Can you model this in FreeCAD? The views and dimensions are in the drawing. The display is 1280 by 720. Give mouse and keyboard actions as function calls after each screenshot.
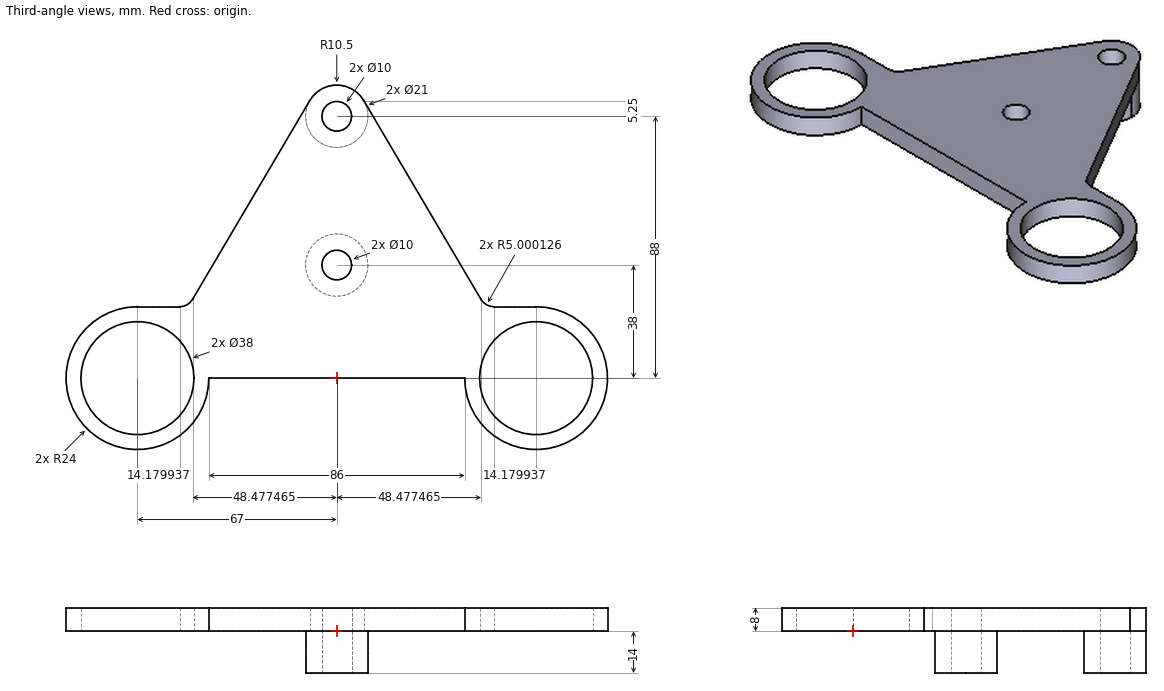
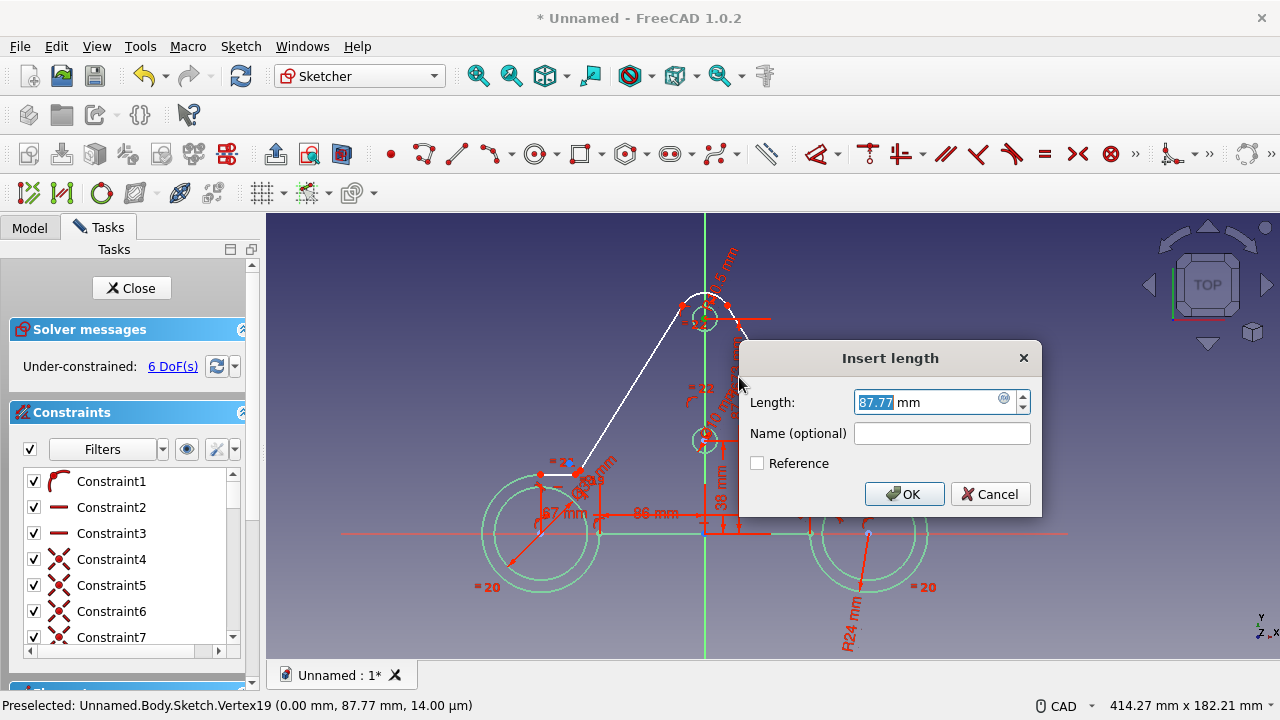
text(88)
key(Return)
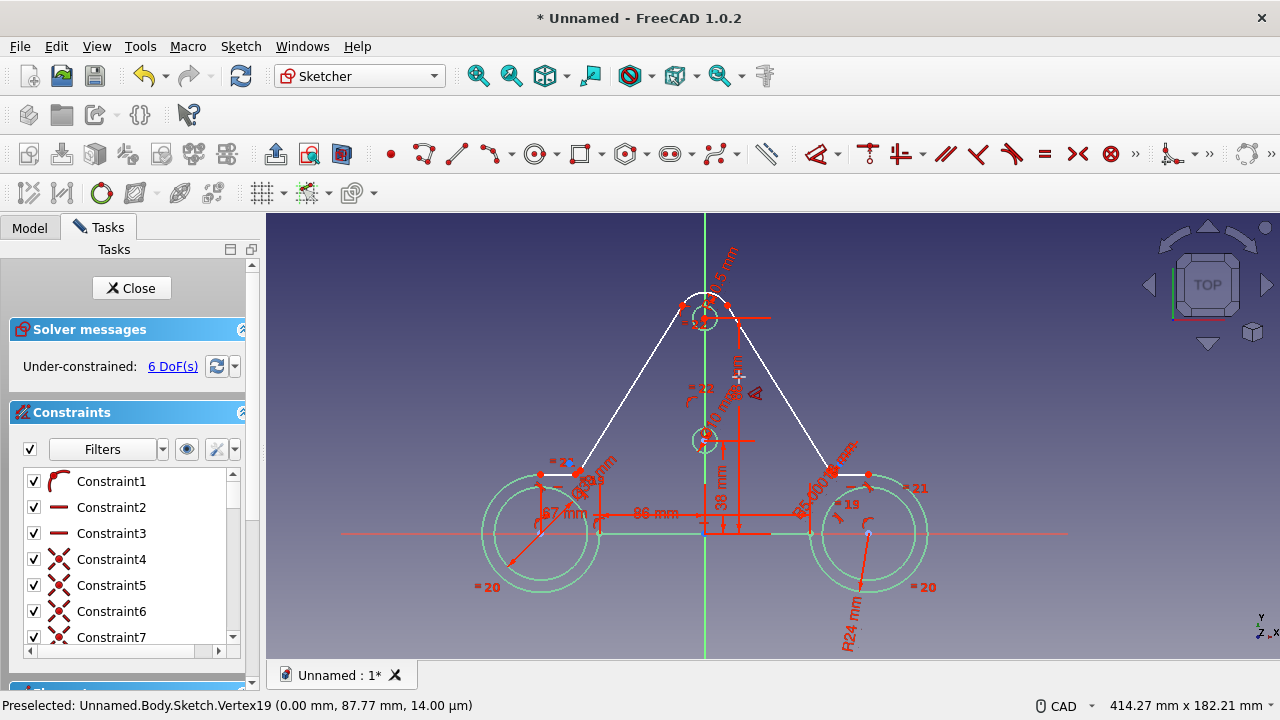
scroll(727, 306, up, 6)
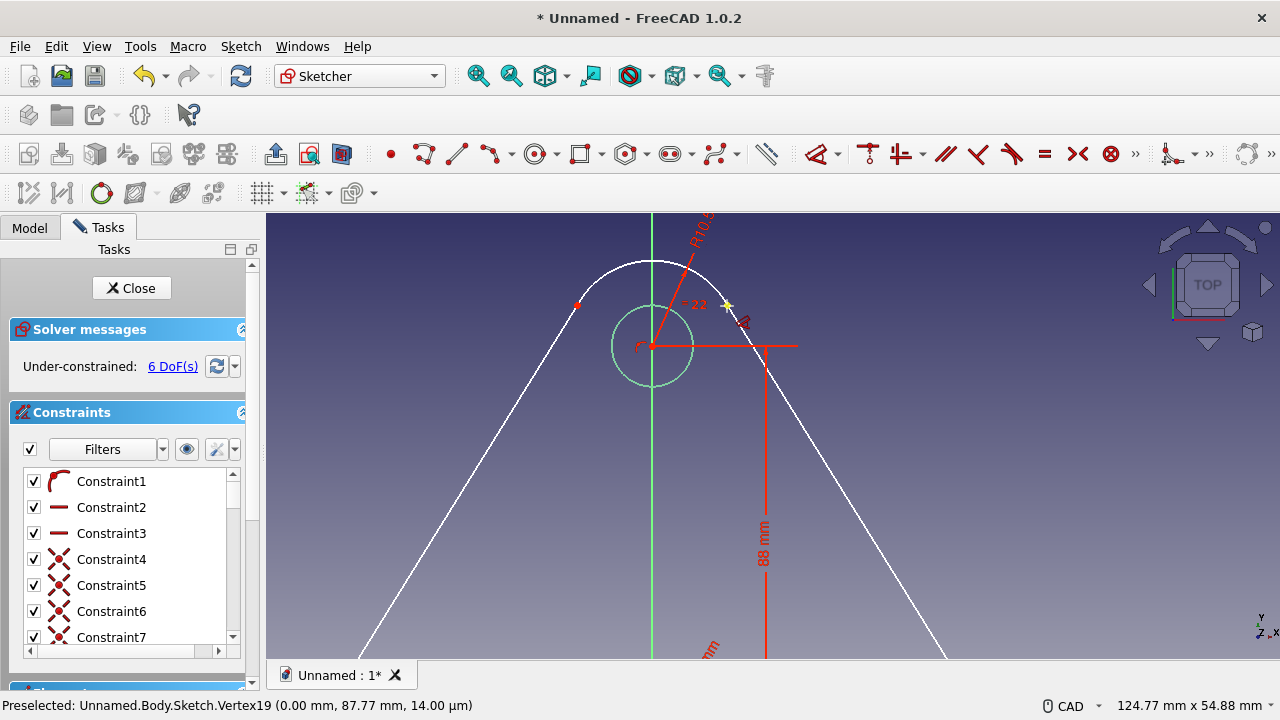
click(727, 305)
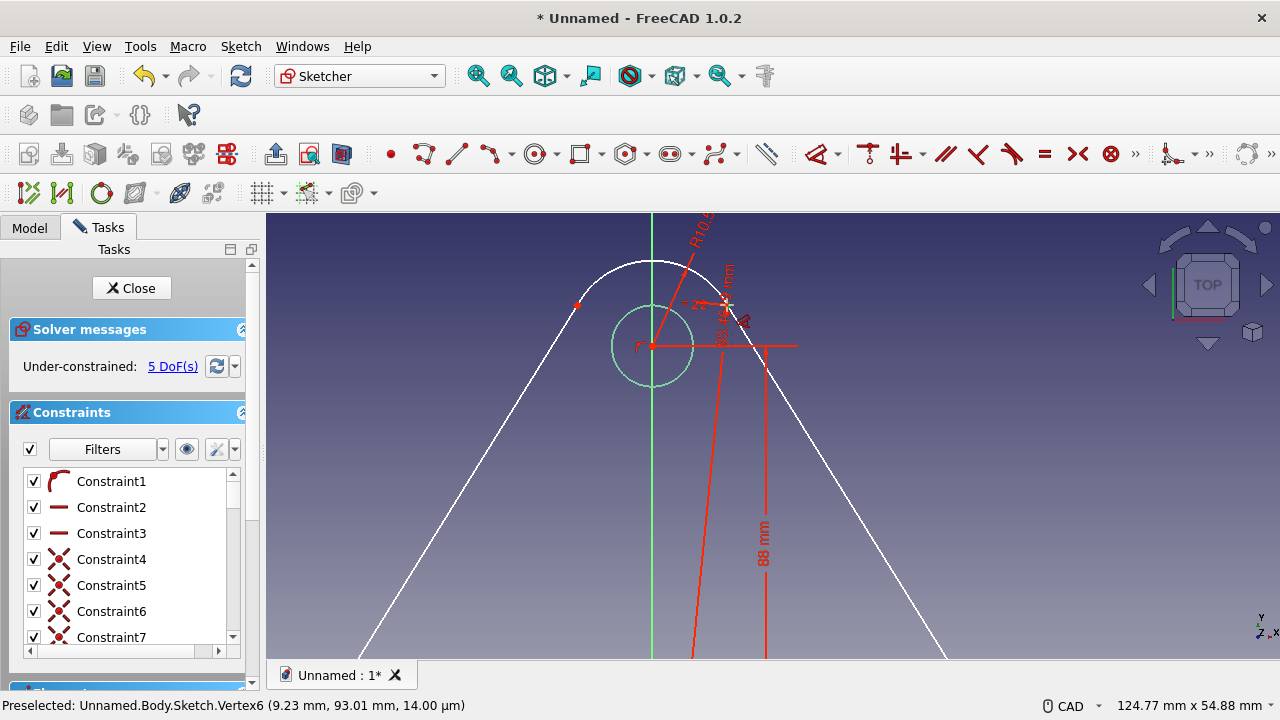
click(652, 346)
click(761, 326)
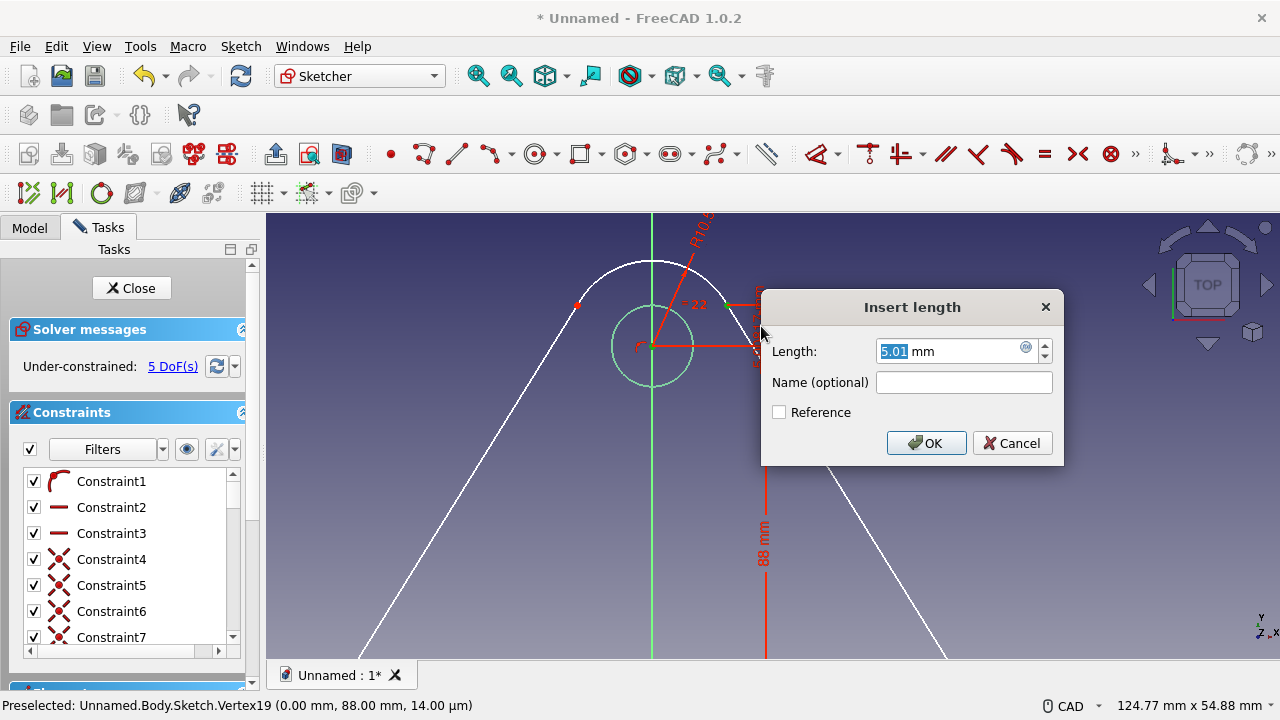
text(5.25)
key(Return)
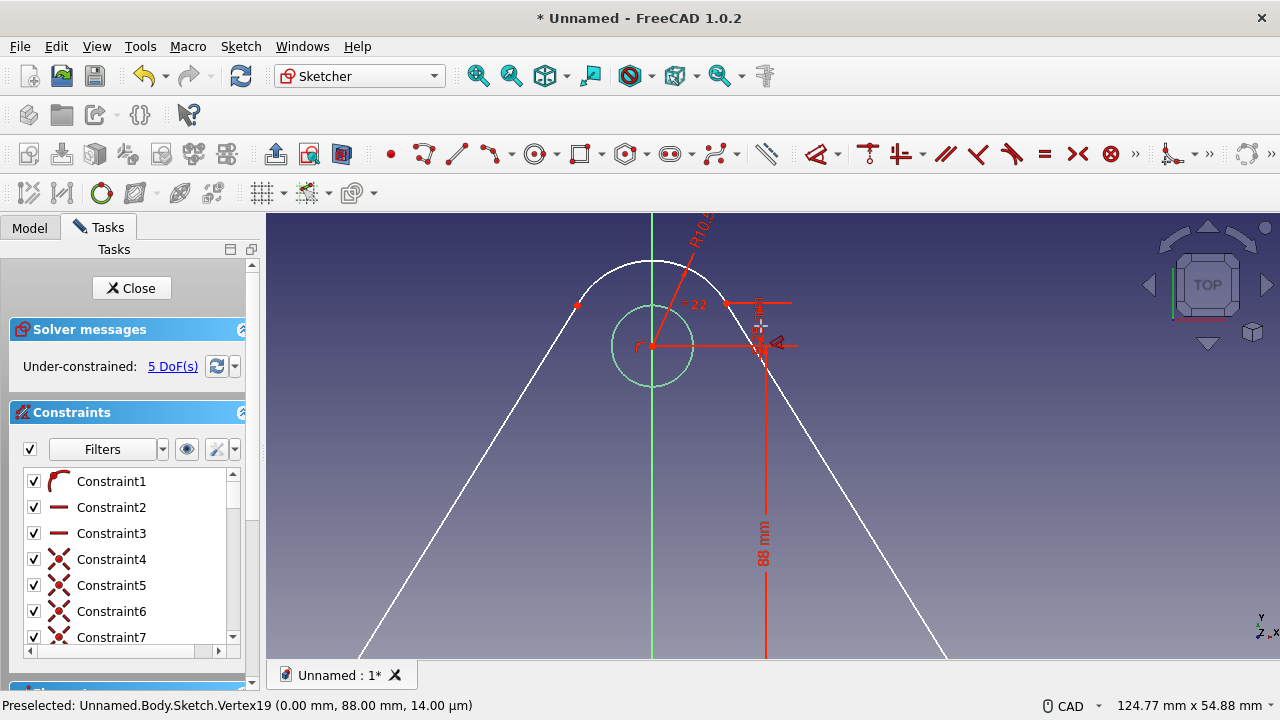
click(577, 305)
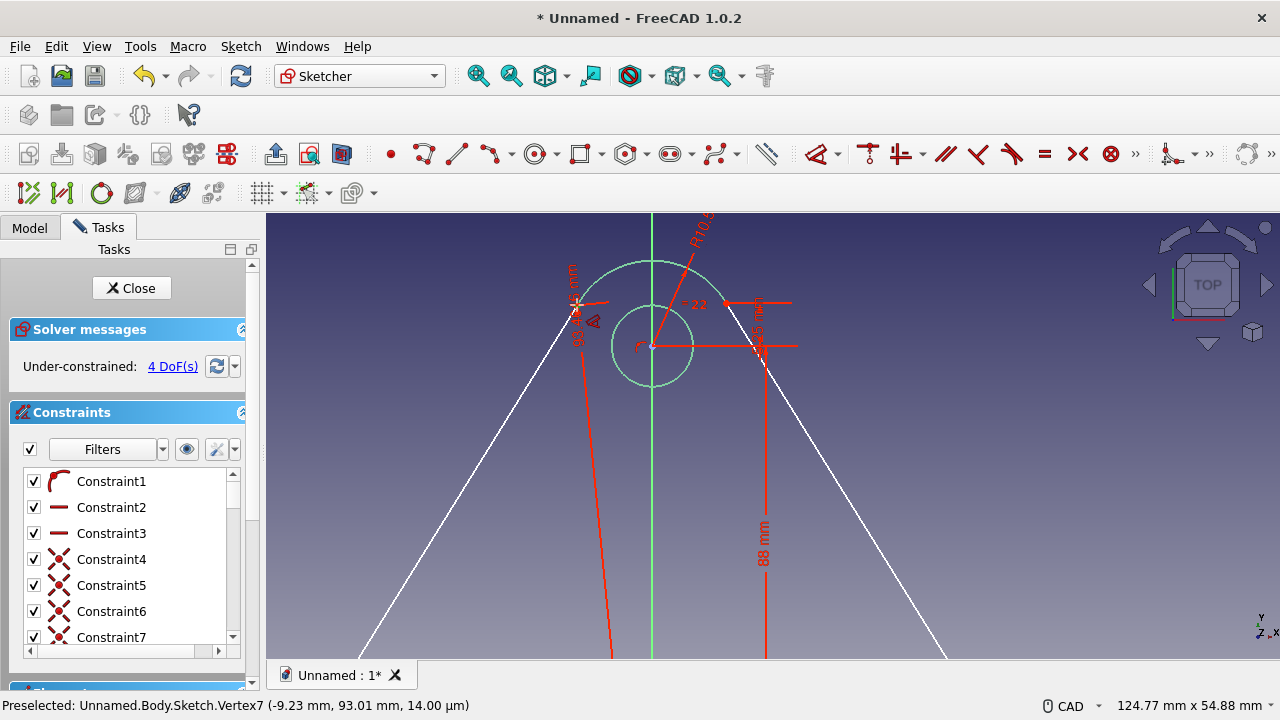
click(652, 346)
click(543, 326)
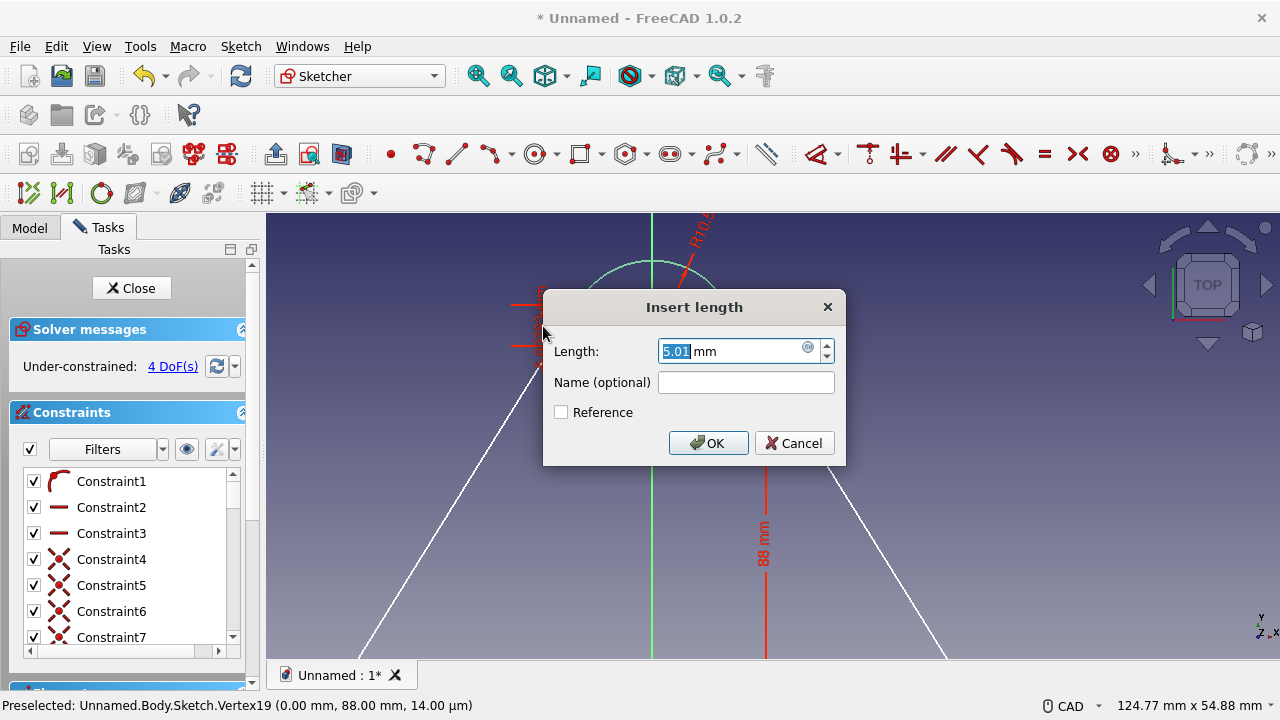
text(5.25)
key(Return)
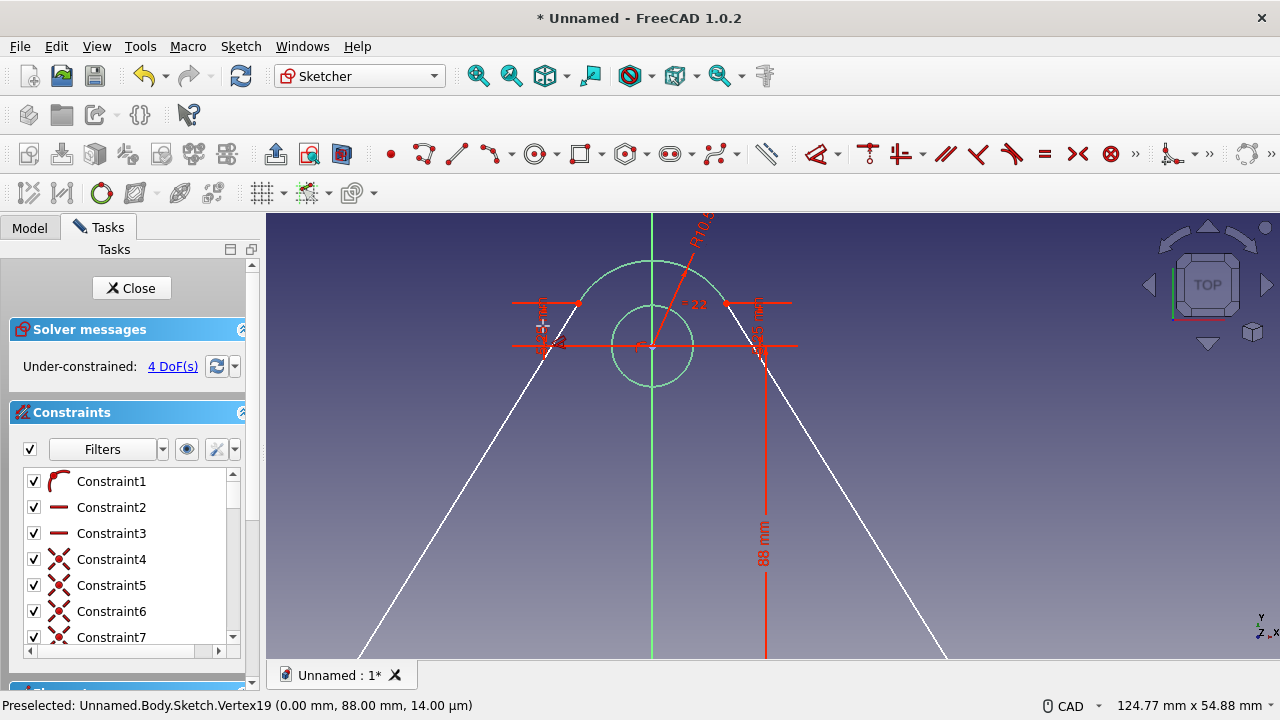
scroll(727, 306, down, 6)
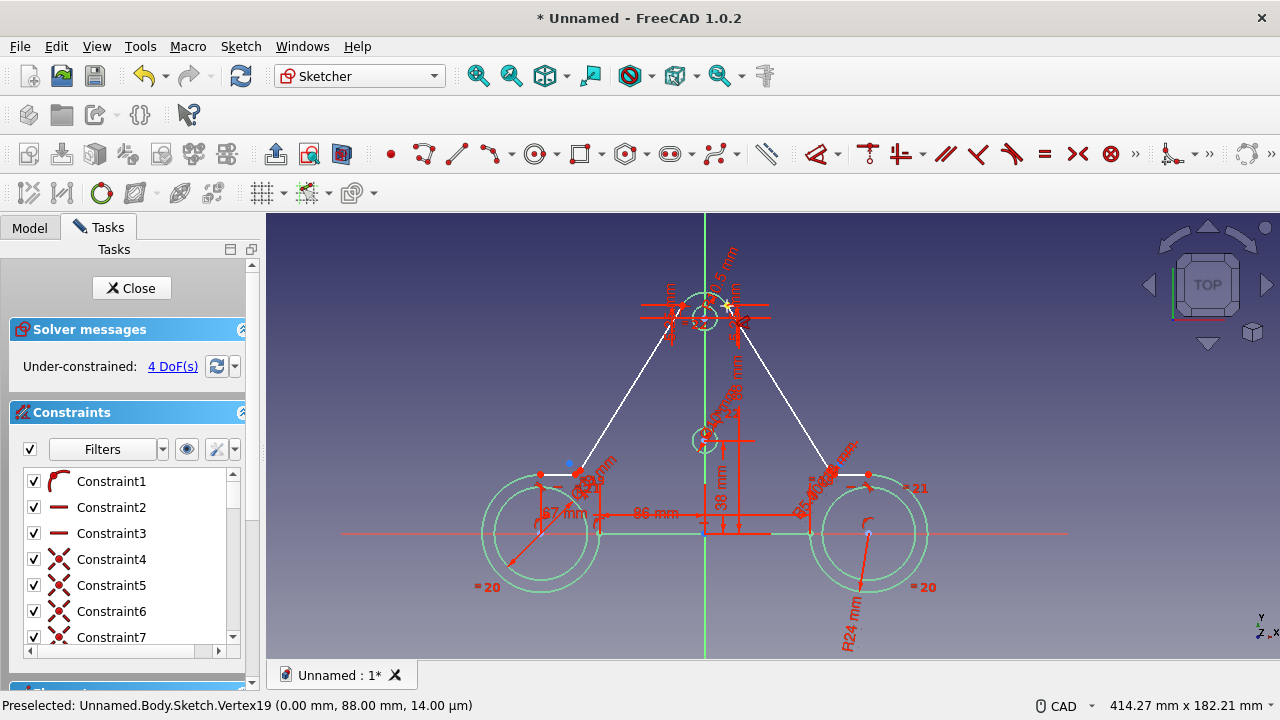
scroll(859, 475, up, 2)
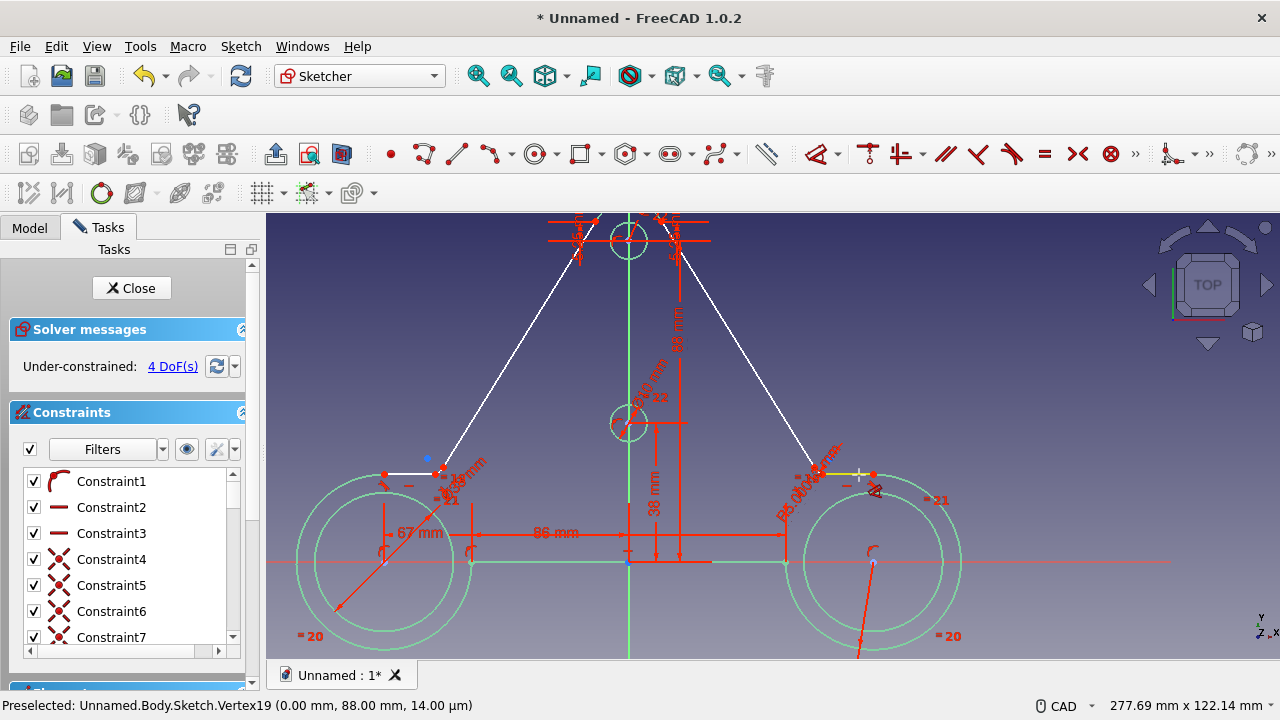
click(858, 474)
click(860, 508)